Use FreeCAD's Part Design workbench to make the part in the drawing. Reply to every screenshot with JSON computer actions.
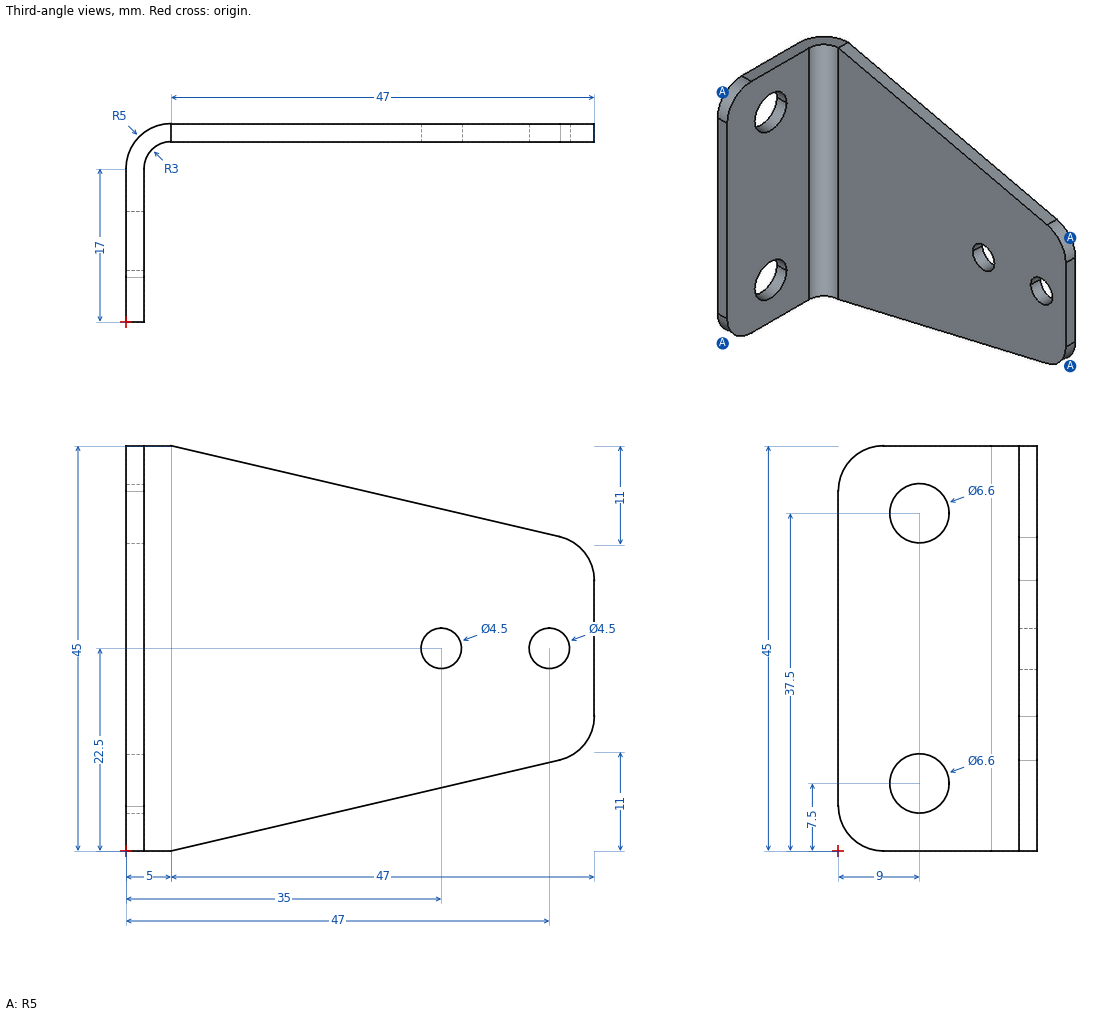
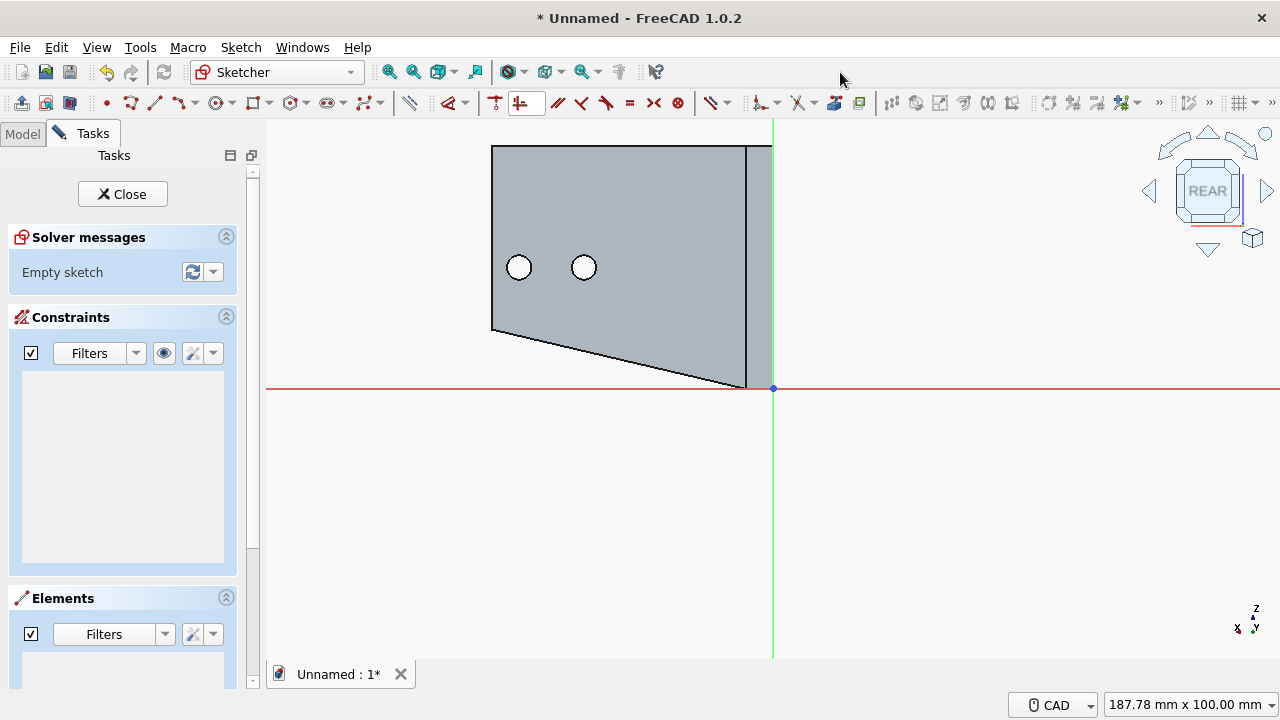
{"action": "scroll", "coordinate": [1029, 631], "scroll_direction": "down", "scroll_amount": 1}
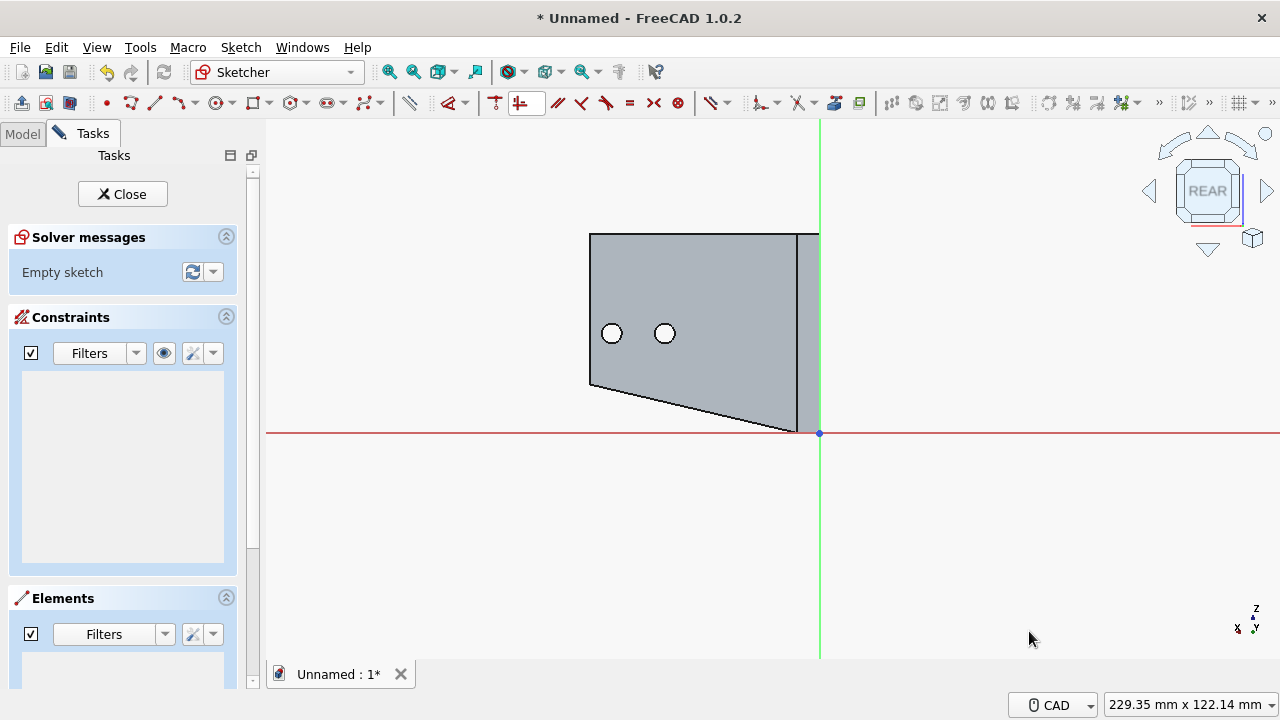
{"action": "scroll", "coordinate": [705, 266], "scroll_direction": "up", "scroll_amount": 3}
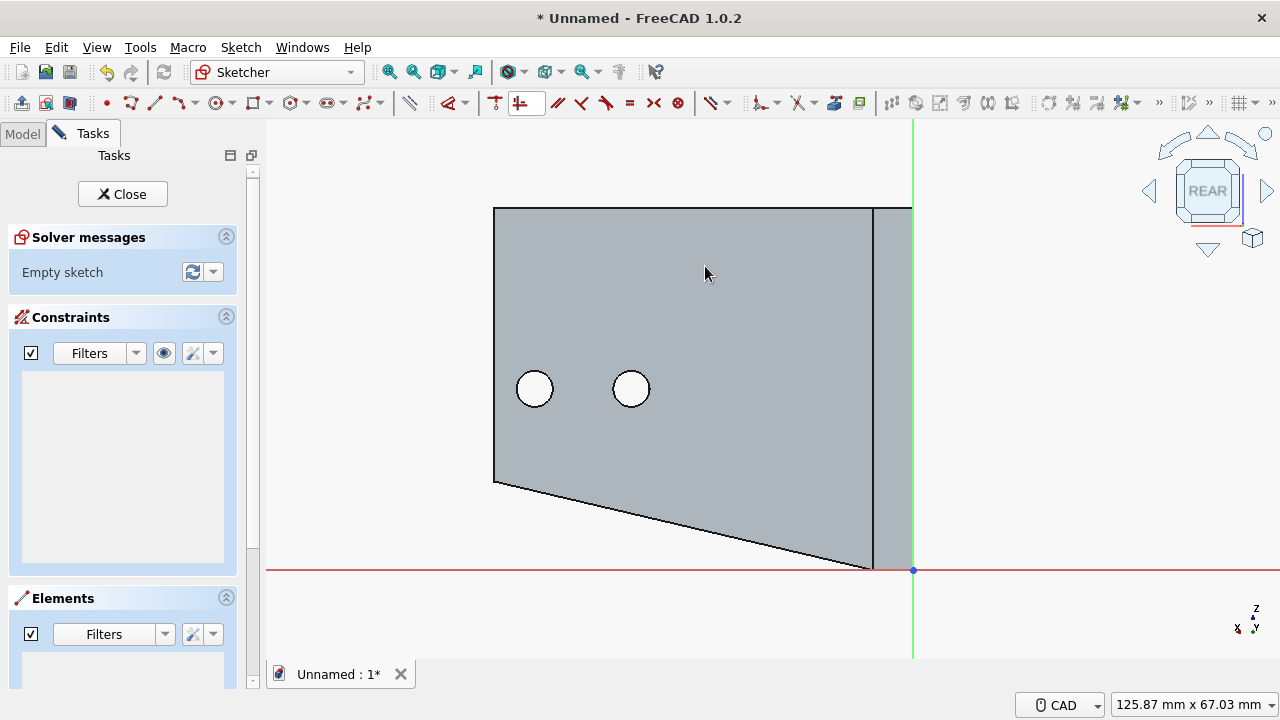
{"action": "key", "text": "g m"}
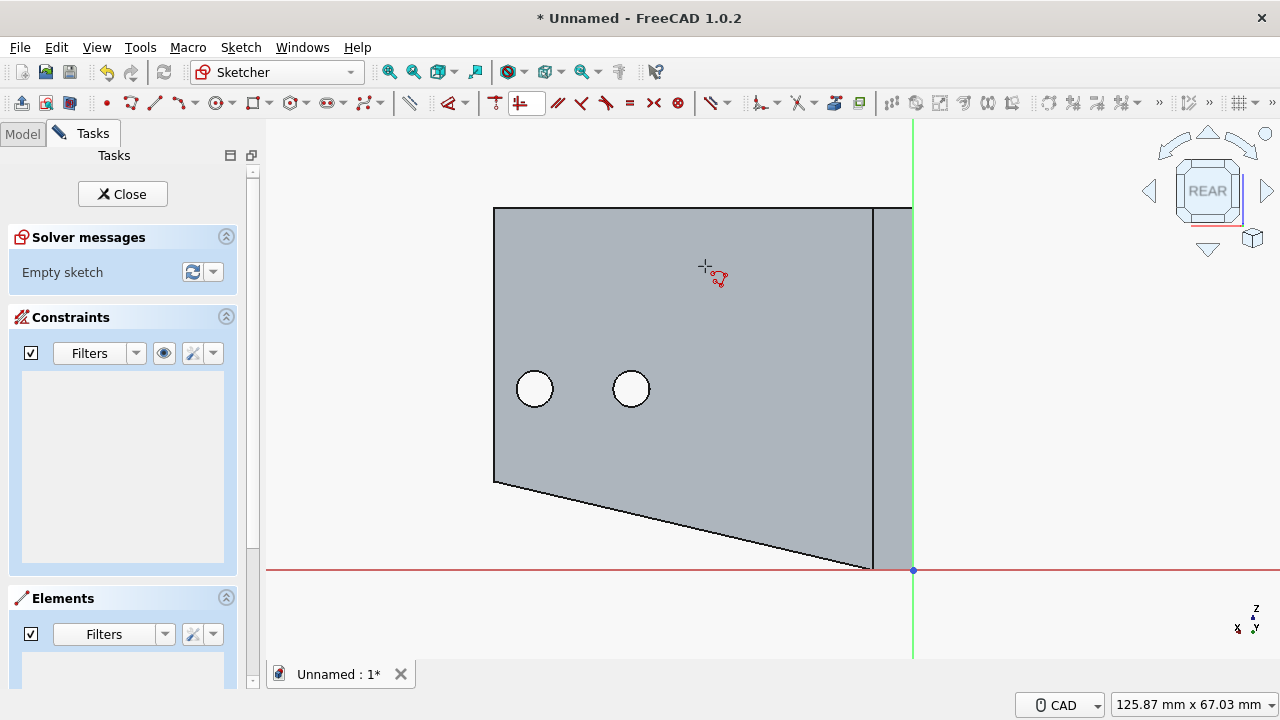
{"action": "left_click", "coordinate": [873, 208]}
{"action": "left_click", "coordinate": [494, 208]}
{"action": "left_click", "coordinate": [494, 296]}
{"action": "left_click", "coordinate": [873, 209]}
{"action": "key", "text": "Escape"}
{"action": "key", "text": "Escape"}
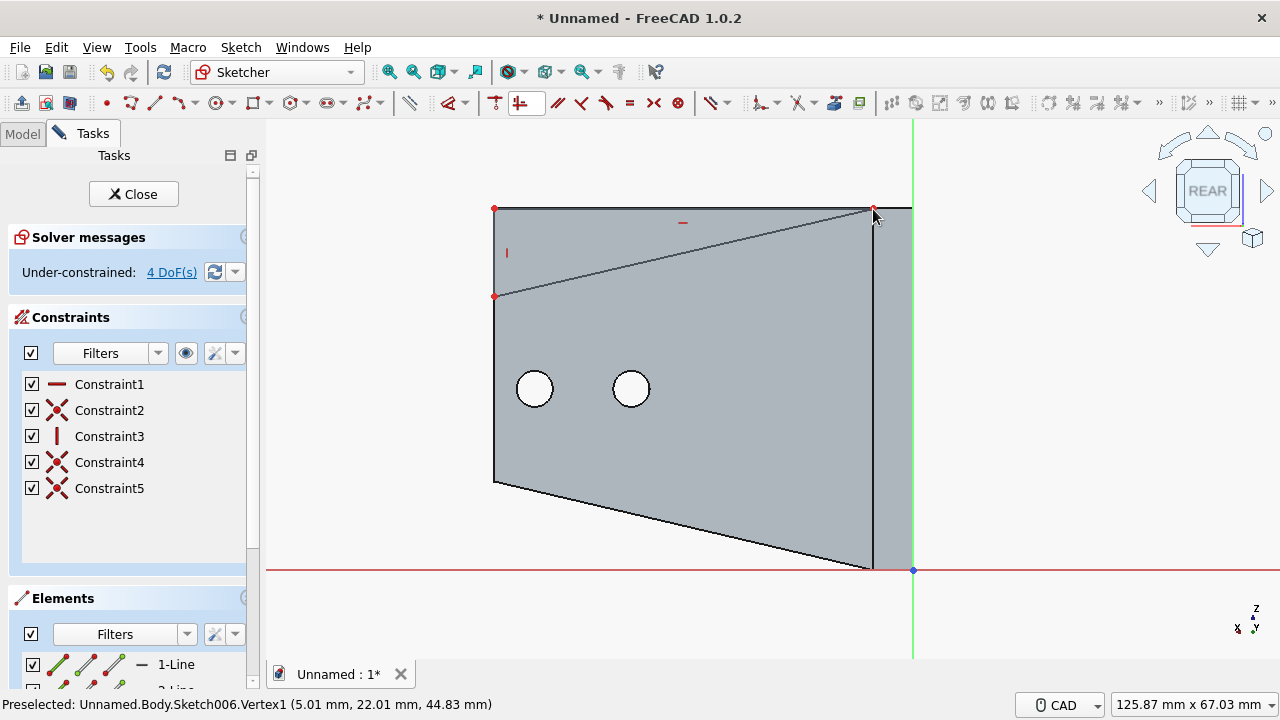
{"action": "key", "text": "d"}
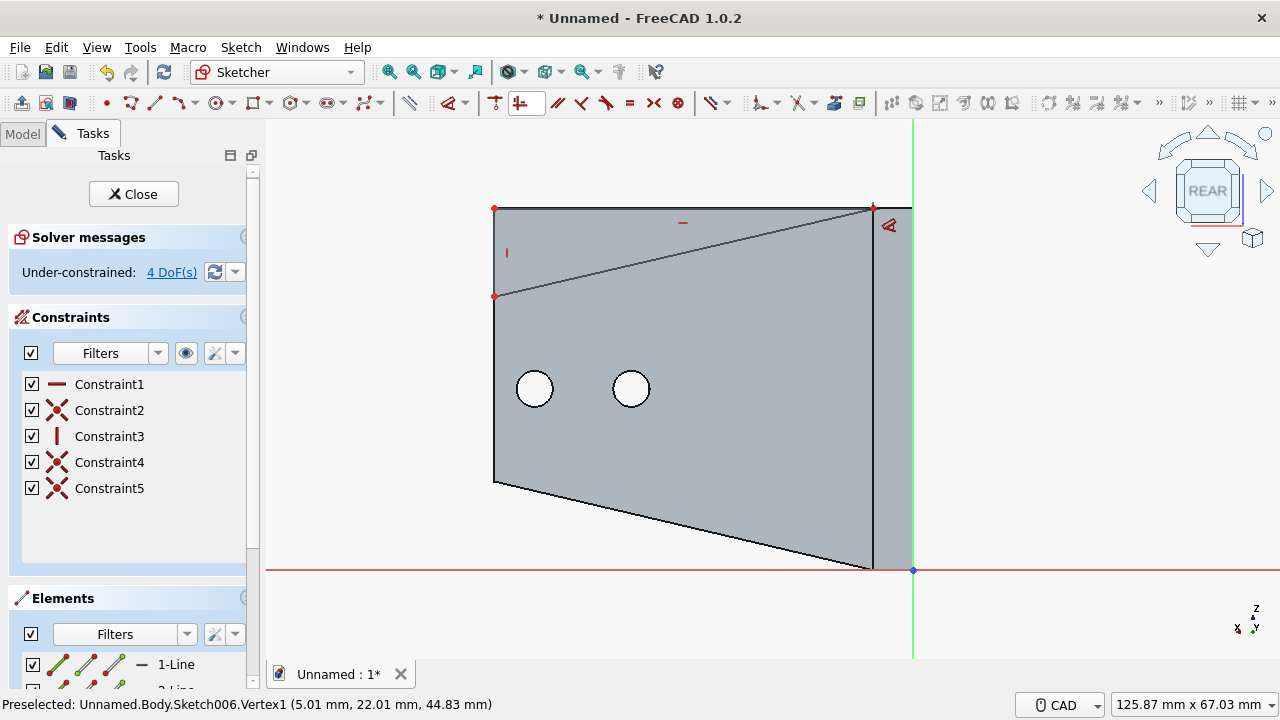
{"action": "left_click", "coordinate": [759, 209]}
{"action": "left_click", "coordinate": [684, 175]}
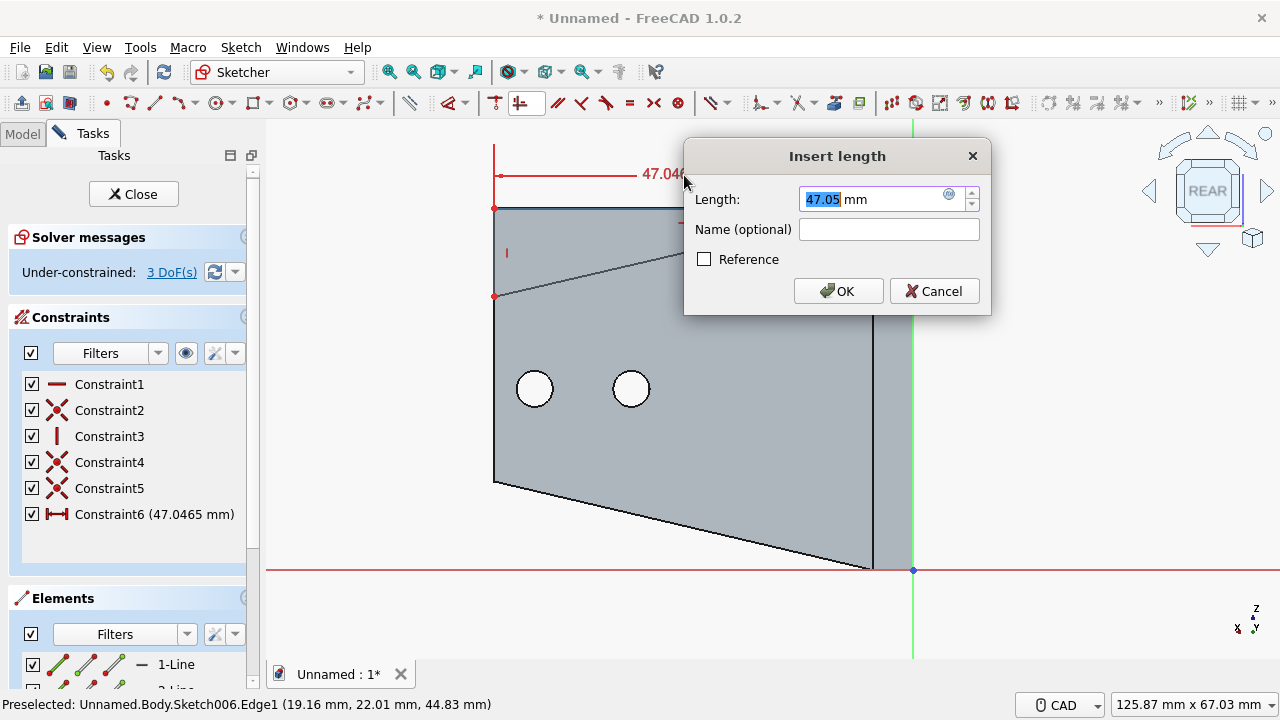
{"action": "type", "text": "47"}
{"action": "key", "text": "Return"}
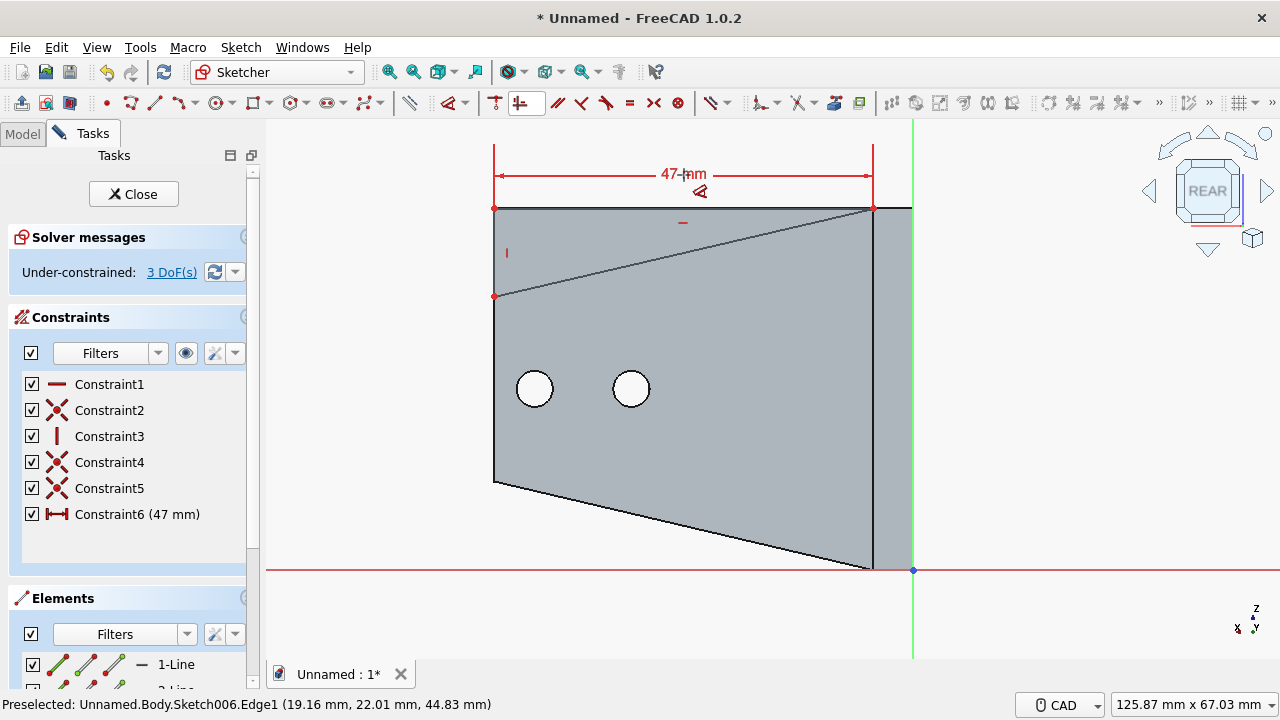
{"action": "left_click", "coordinate": [494, 235]}
{"action": "left_click", "coordinate": [460, 253]}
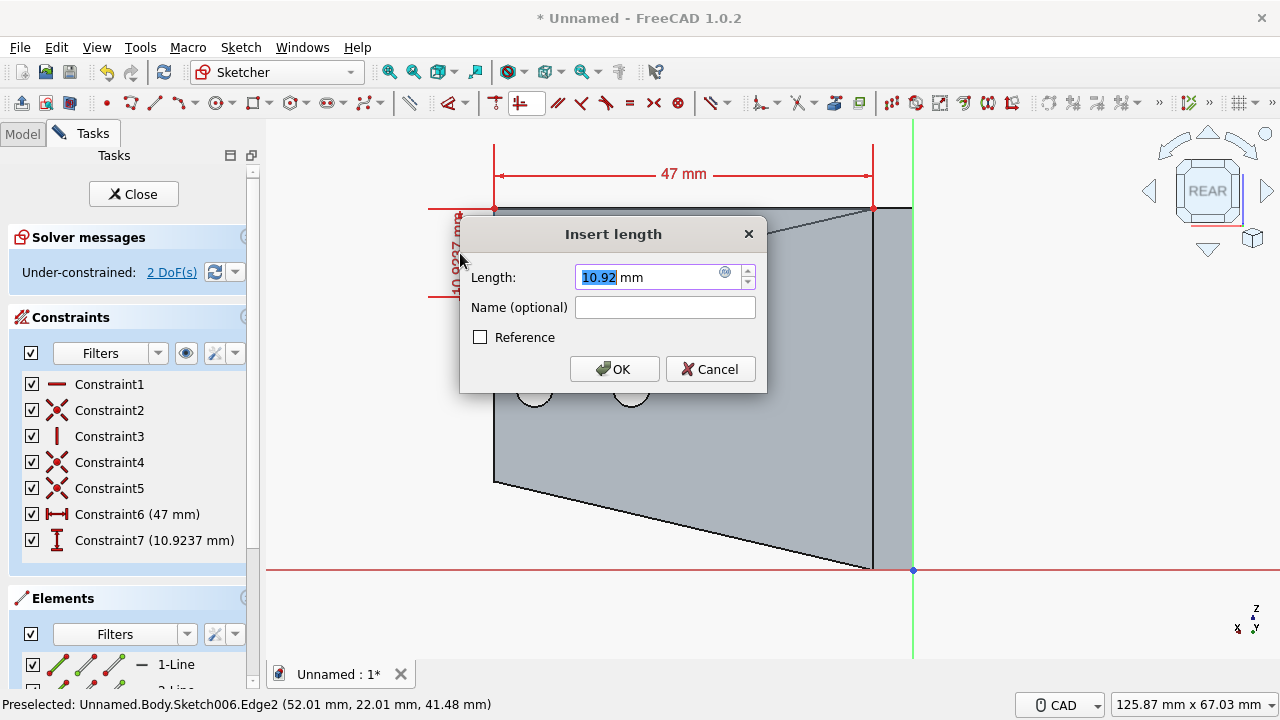
{"action": "type", "text": "11"}
{"action": "key", "text": "Return"}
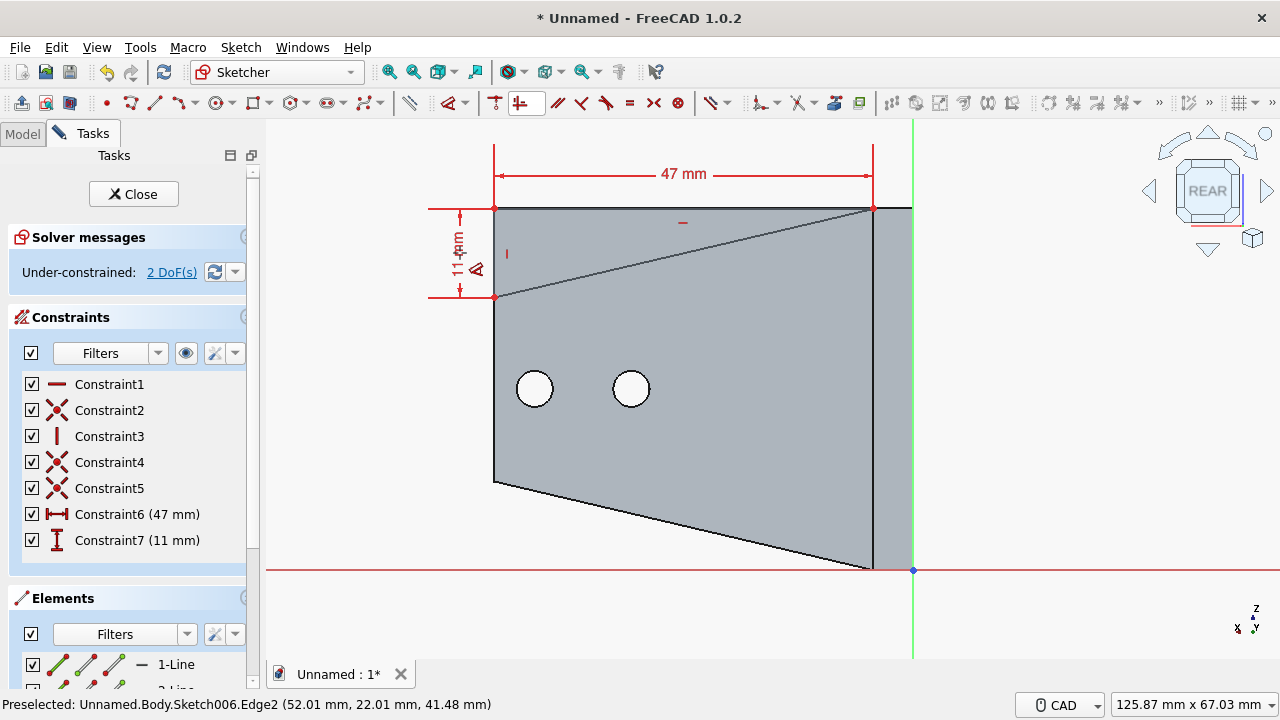
{"action": "left_click", "coordinate": [873, 209]}
{"action": "left_click", "coordinate": [893, 604]}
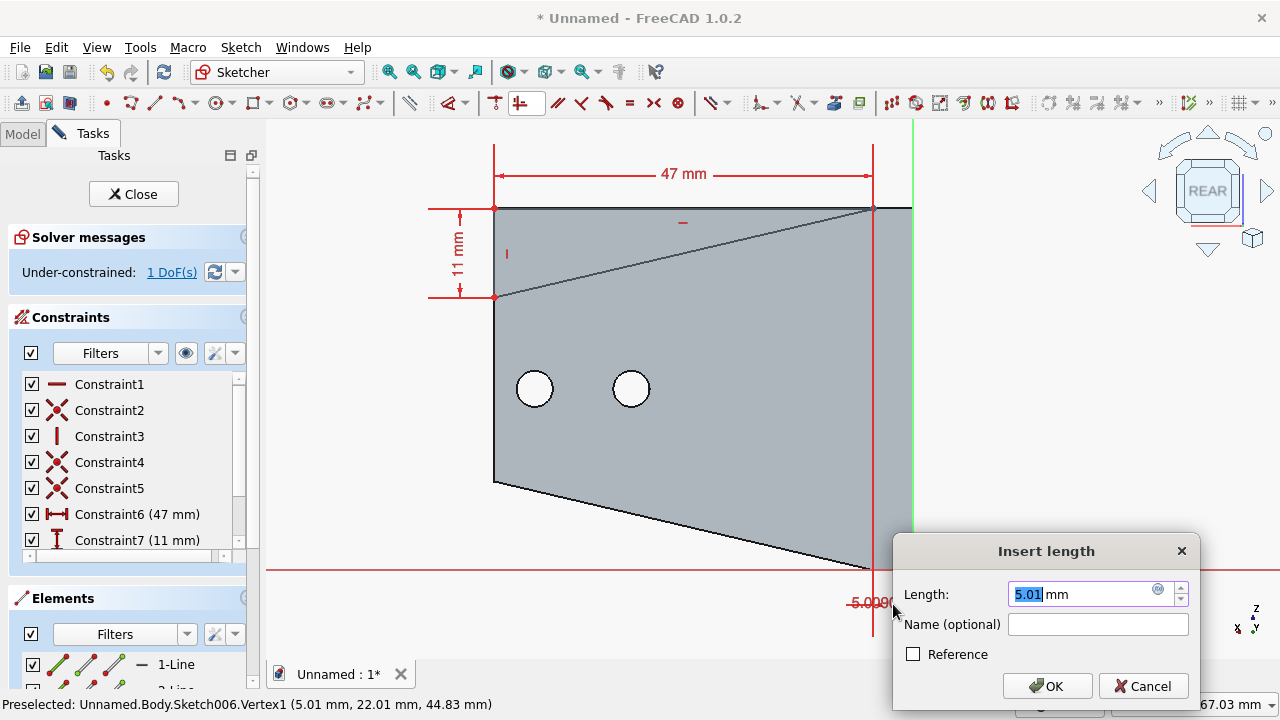
{"action": "type", "text": "5"}
{"action": "key", "text": "Return"}